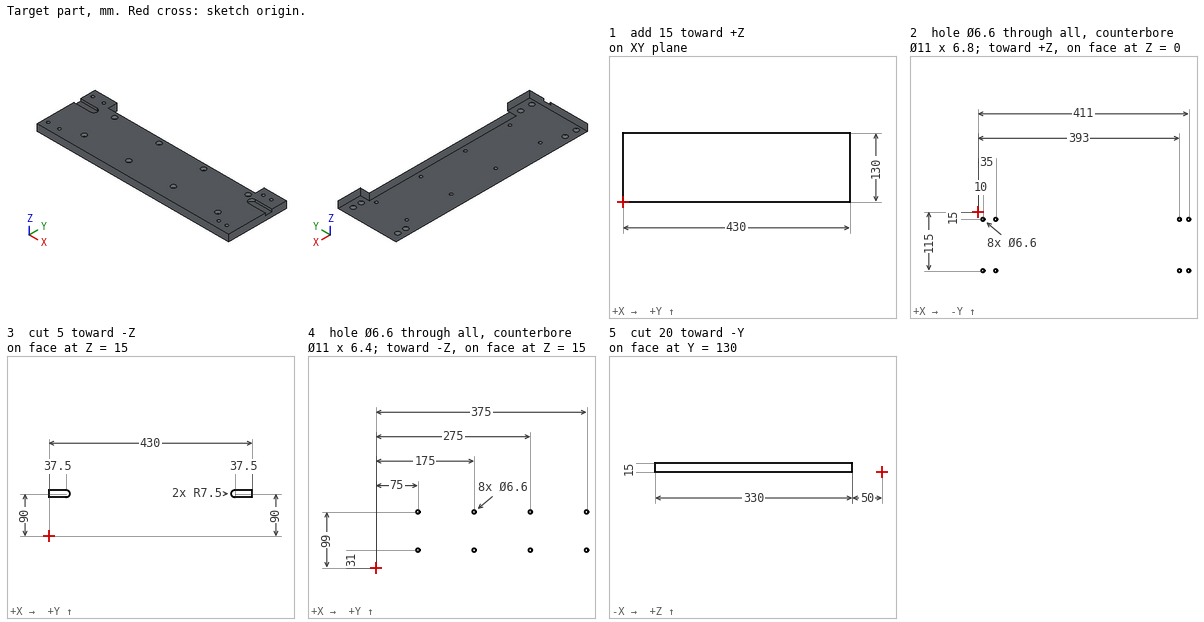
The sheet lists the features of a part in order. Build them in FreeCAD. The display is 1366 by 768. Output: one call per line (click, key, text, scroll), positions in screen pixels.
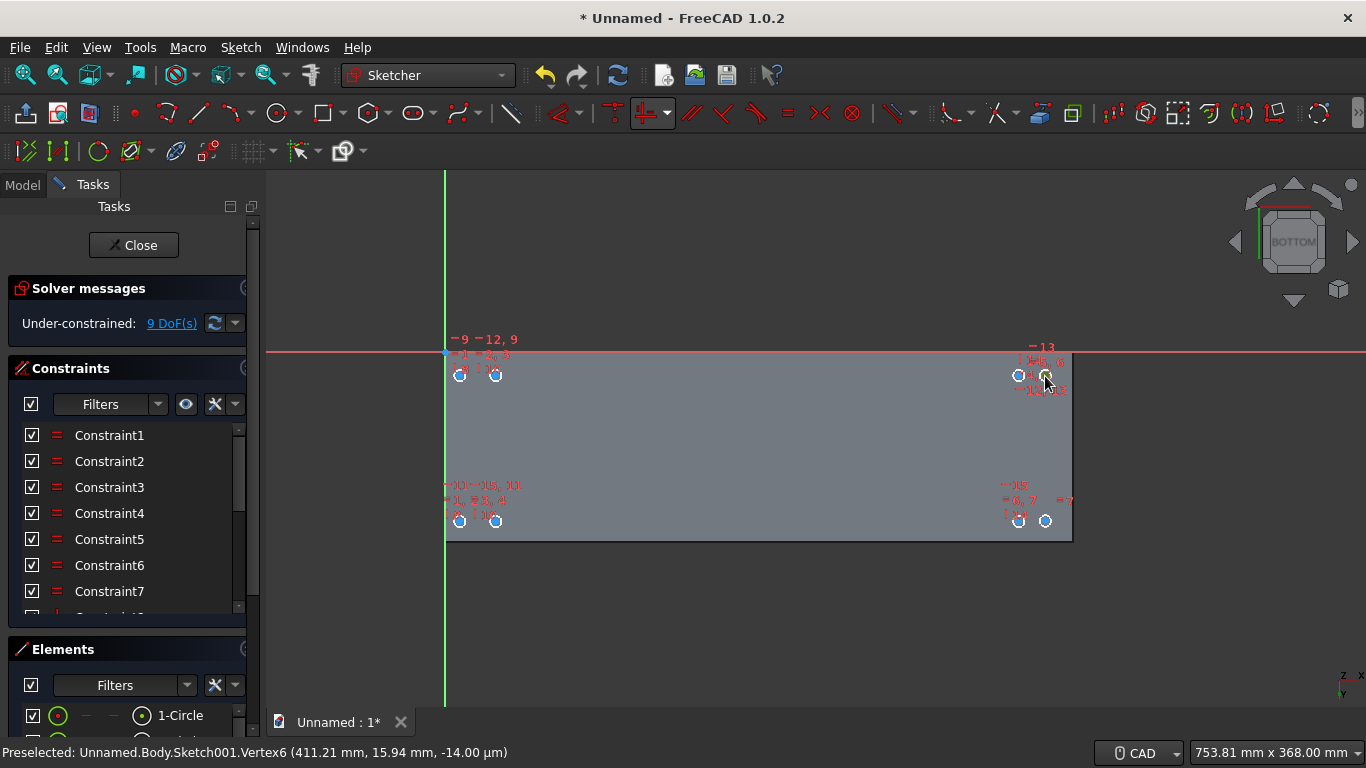
click(1045, 521)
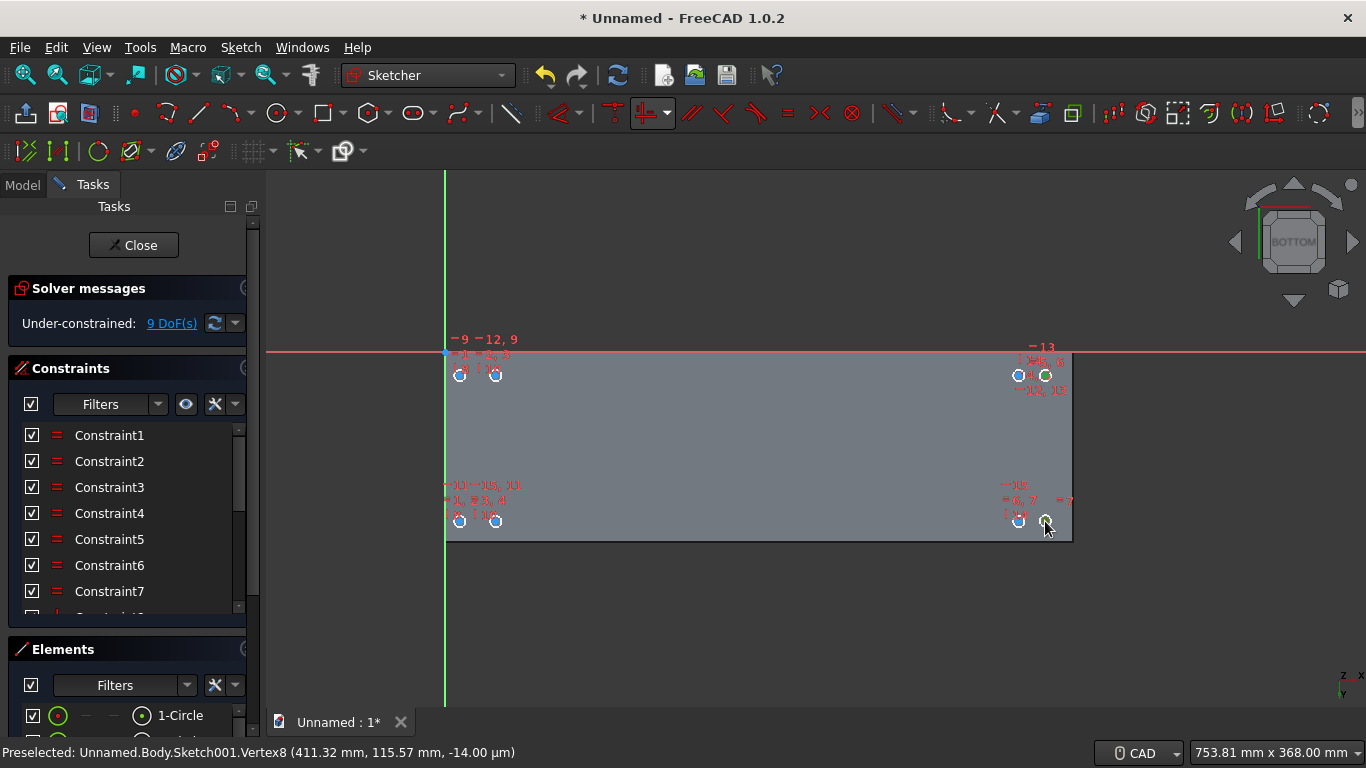
key(v)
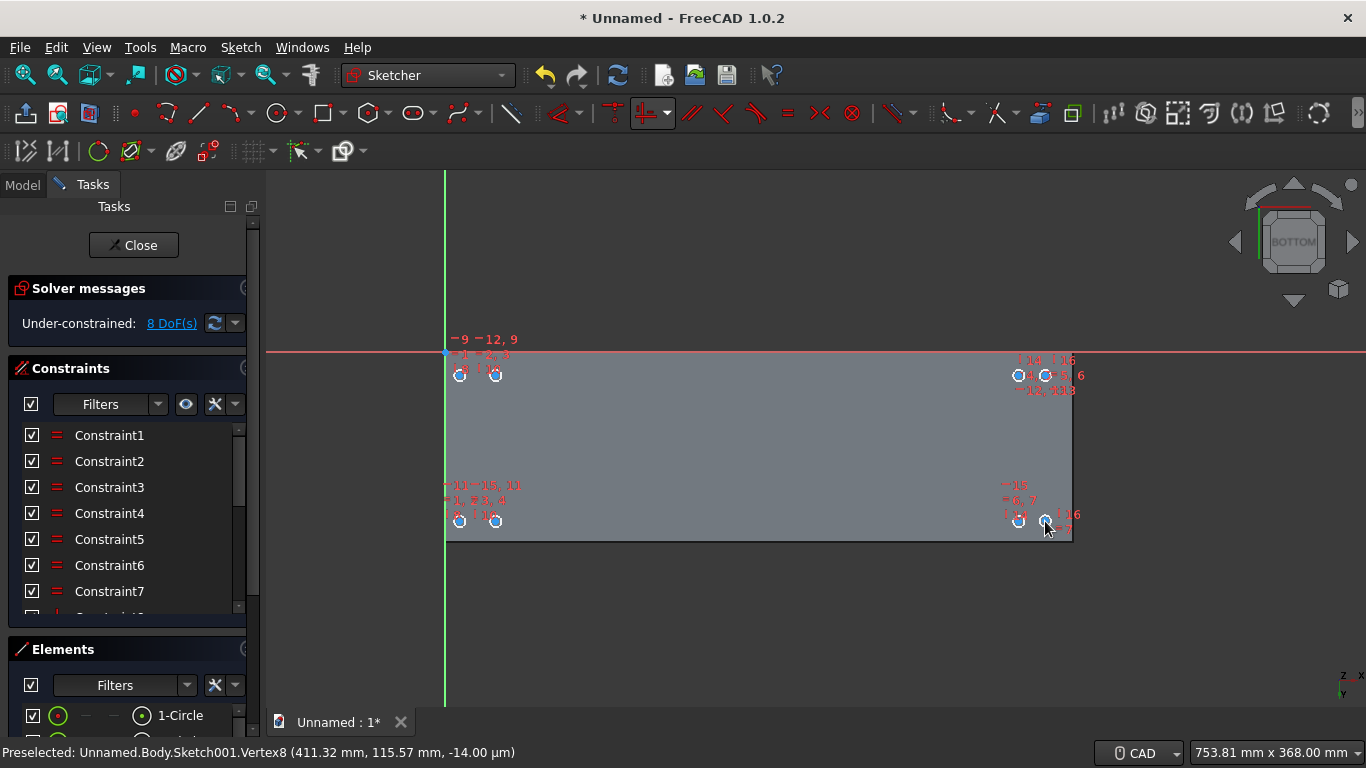
click(1019, 522)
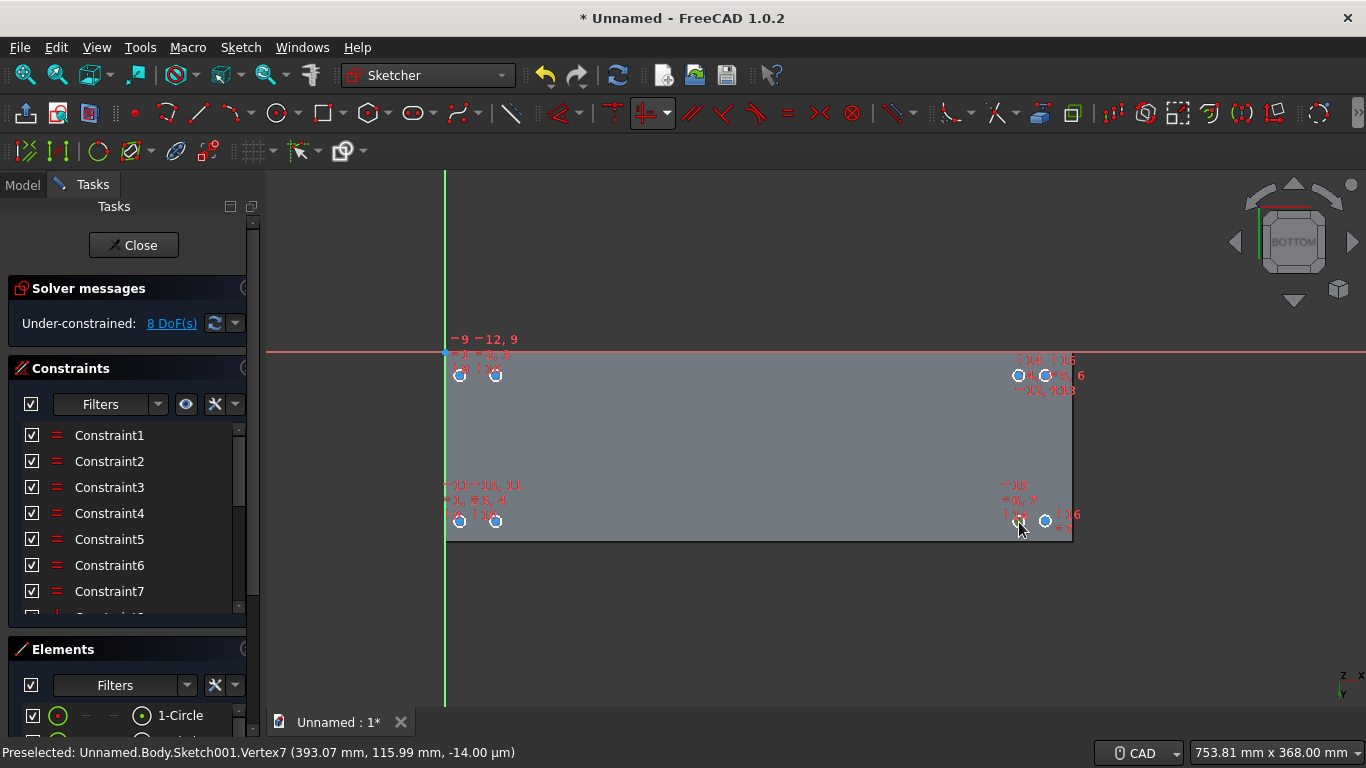
click(1045, 521)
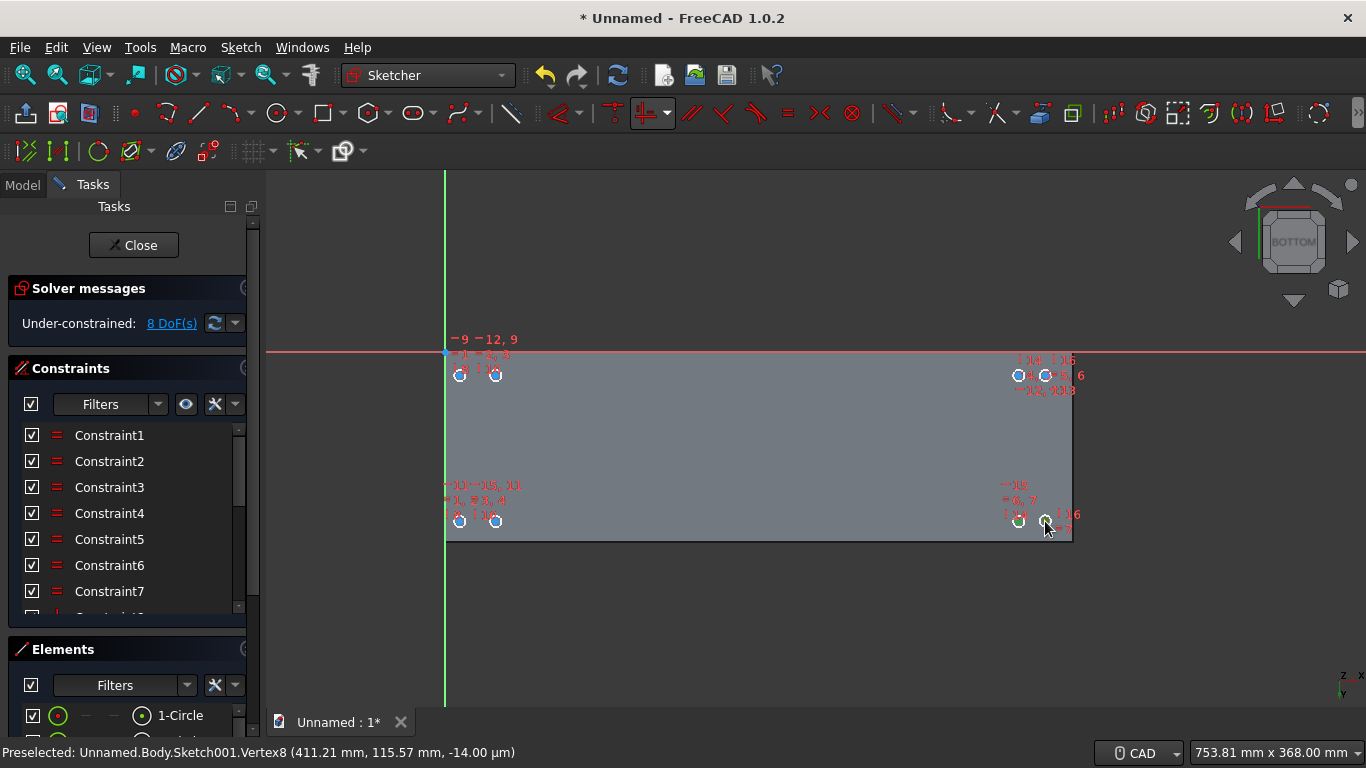
key(h)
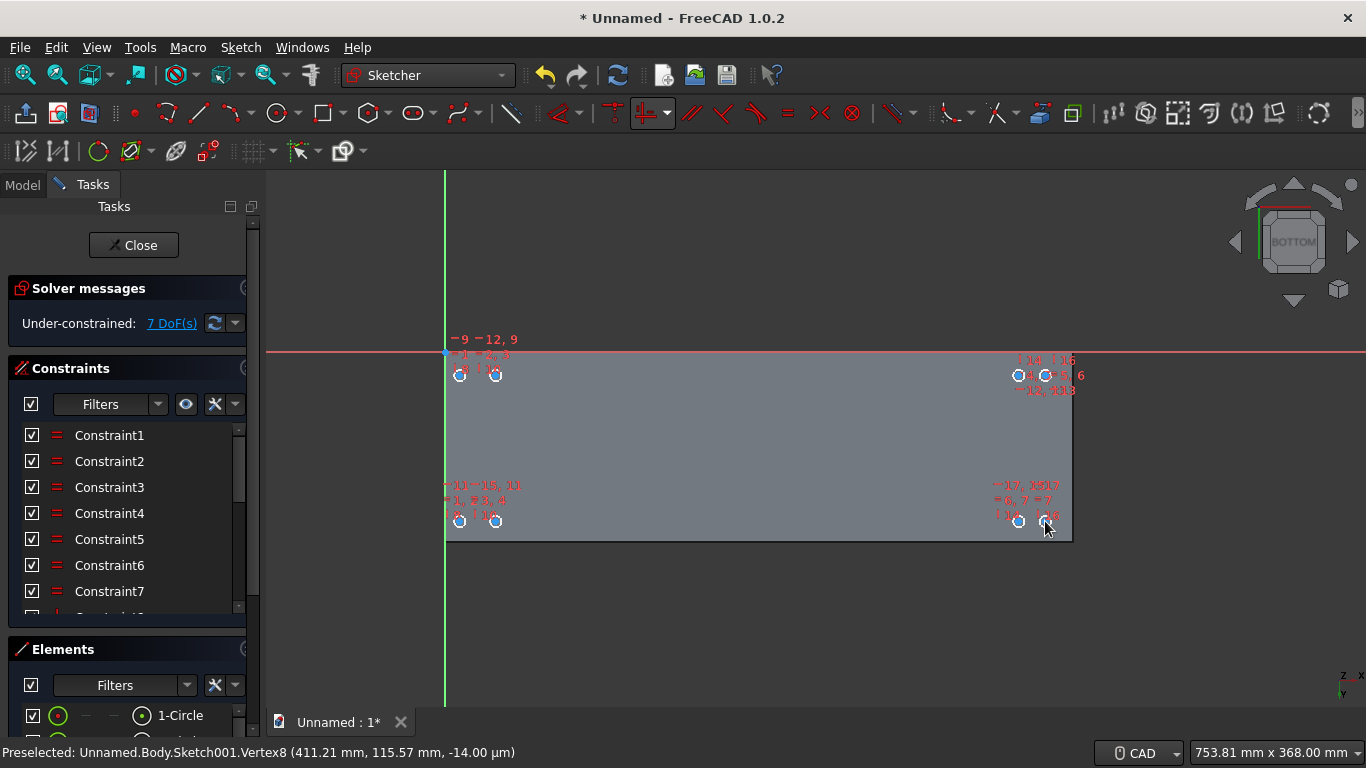
scroll(460, 381, up, 8)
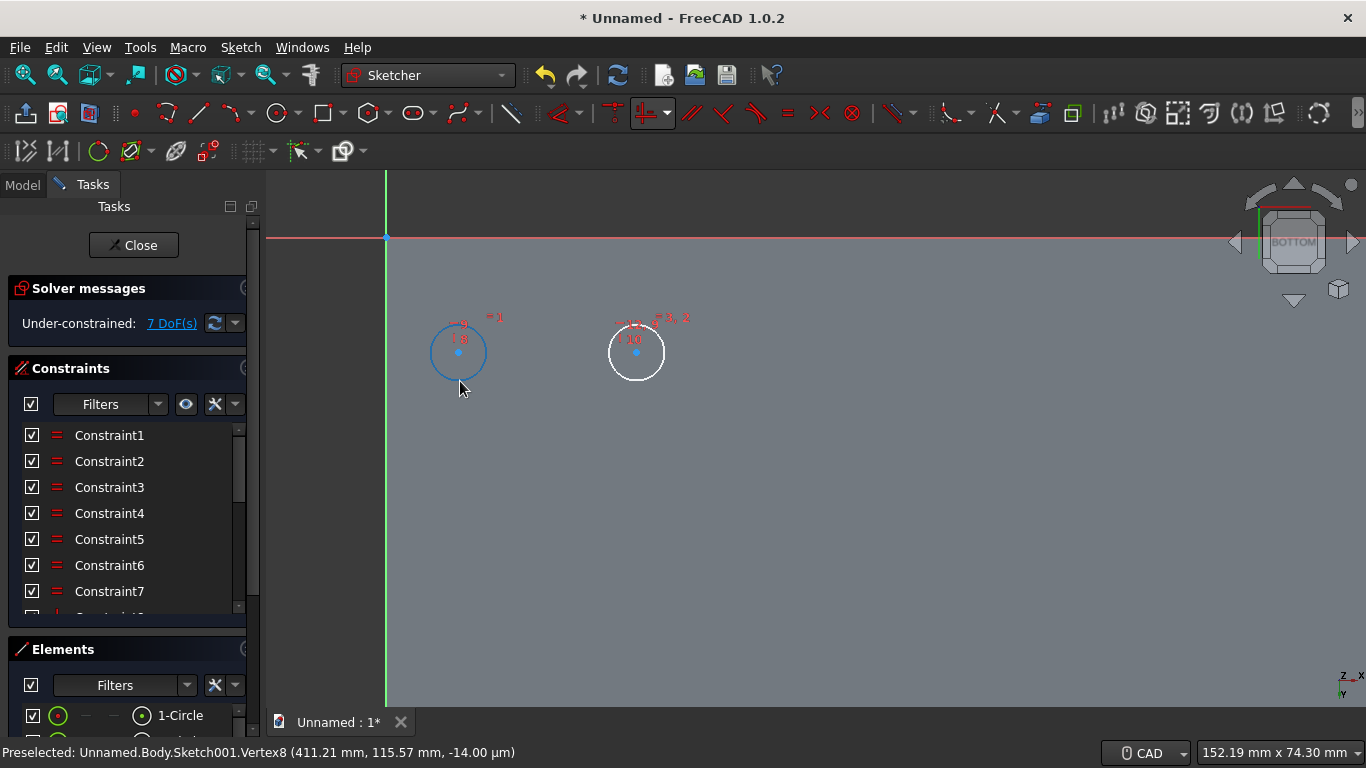
click(458, 381)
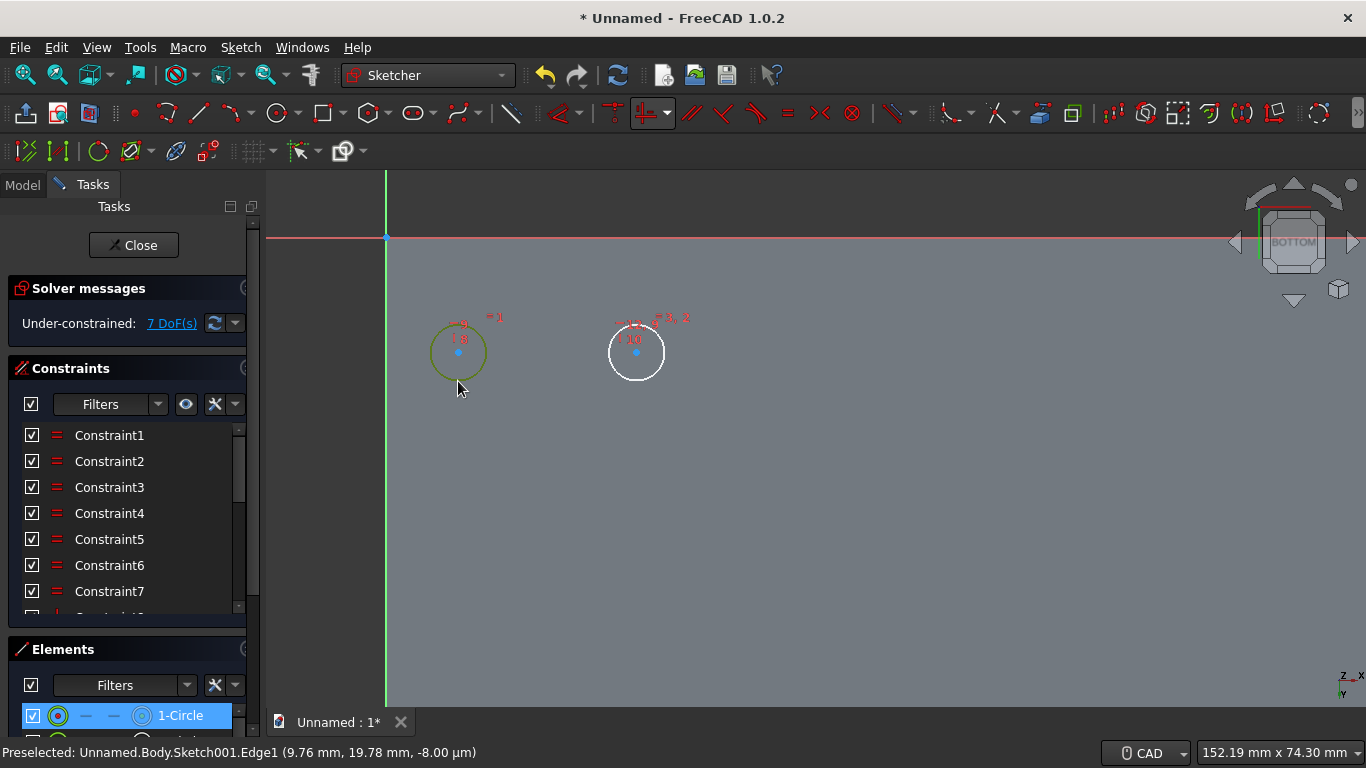
key(k)
key(o)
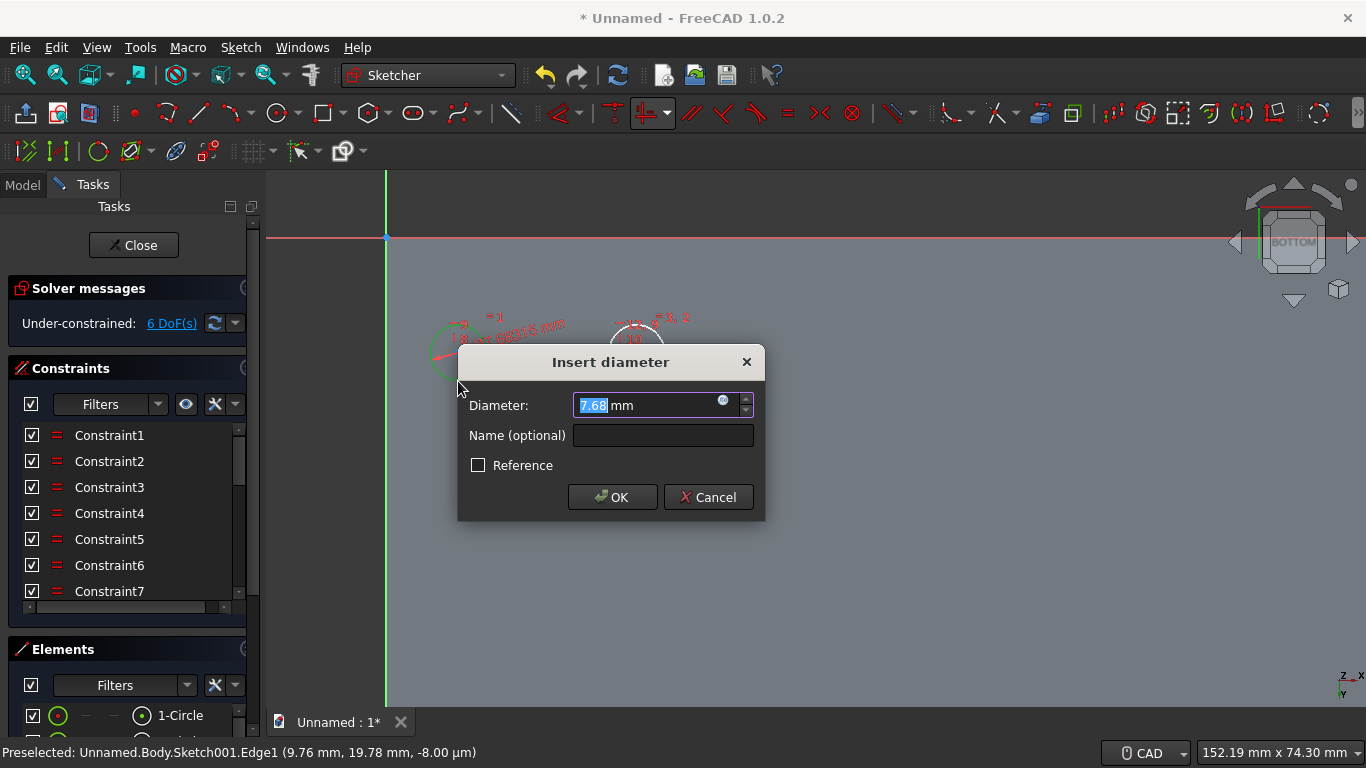
text(6.6)
key(Return)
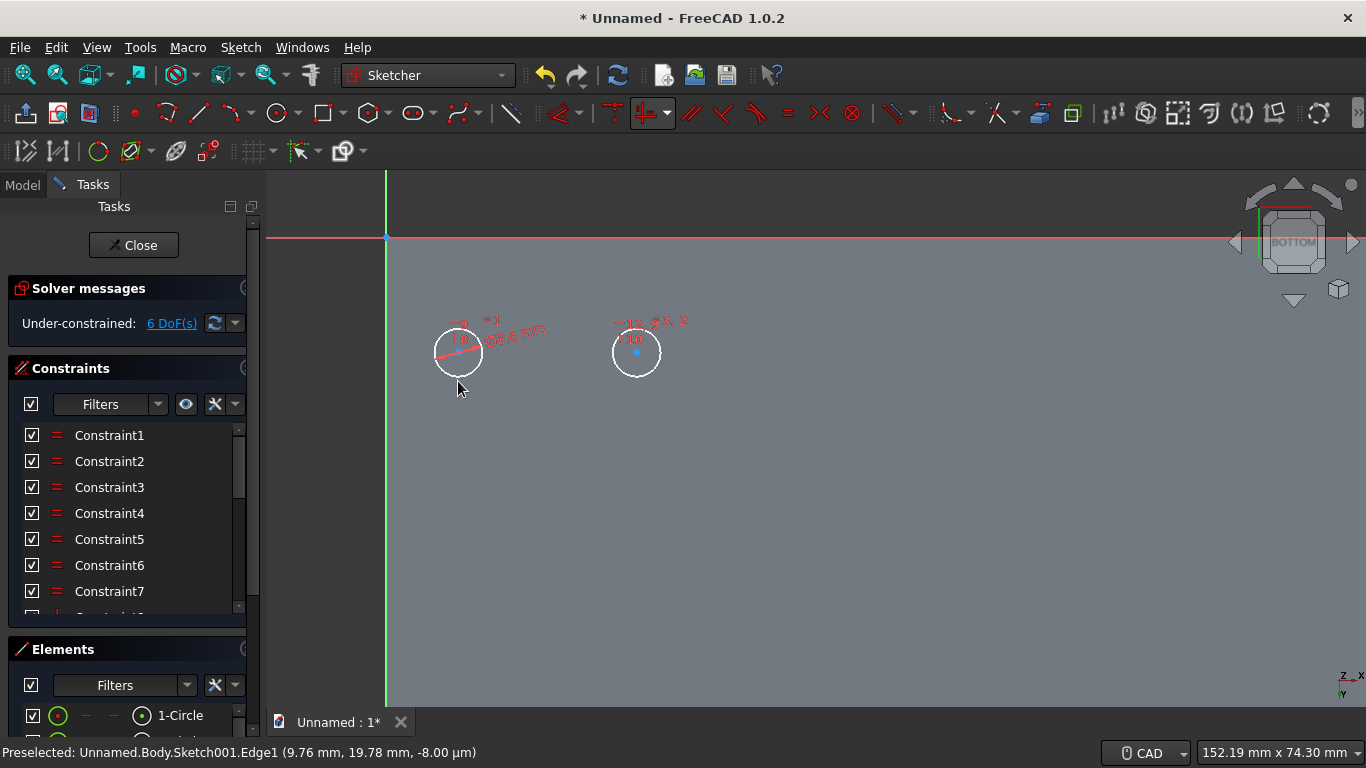
click(458, 353)